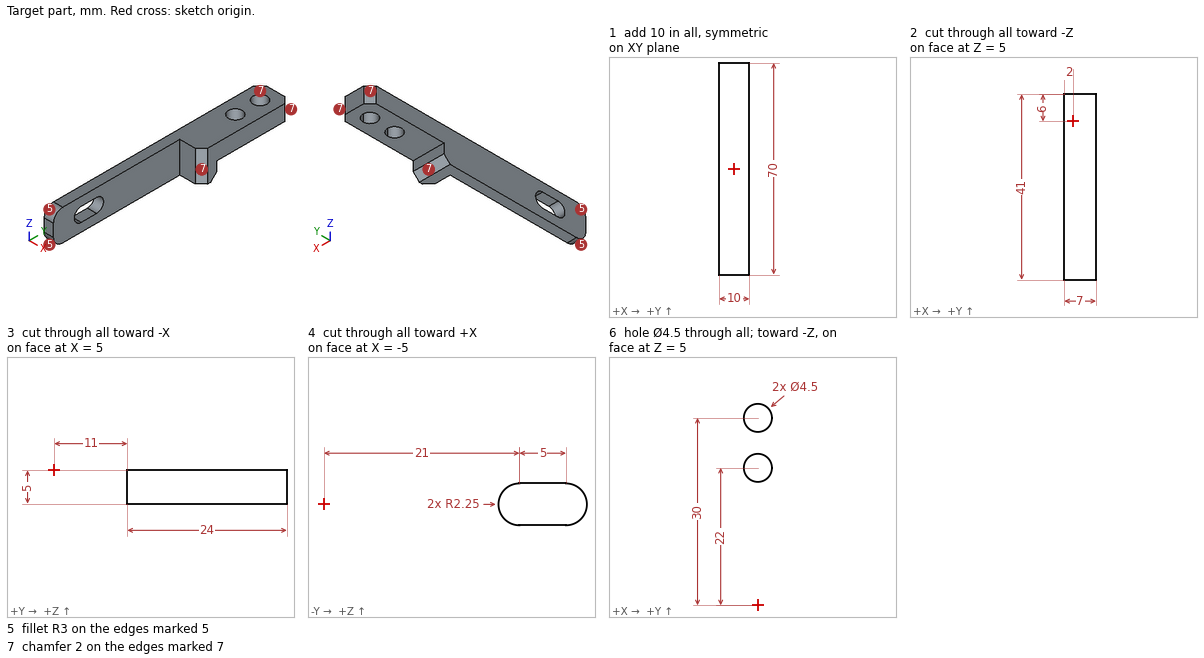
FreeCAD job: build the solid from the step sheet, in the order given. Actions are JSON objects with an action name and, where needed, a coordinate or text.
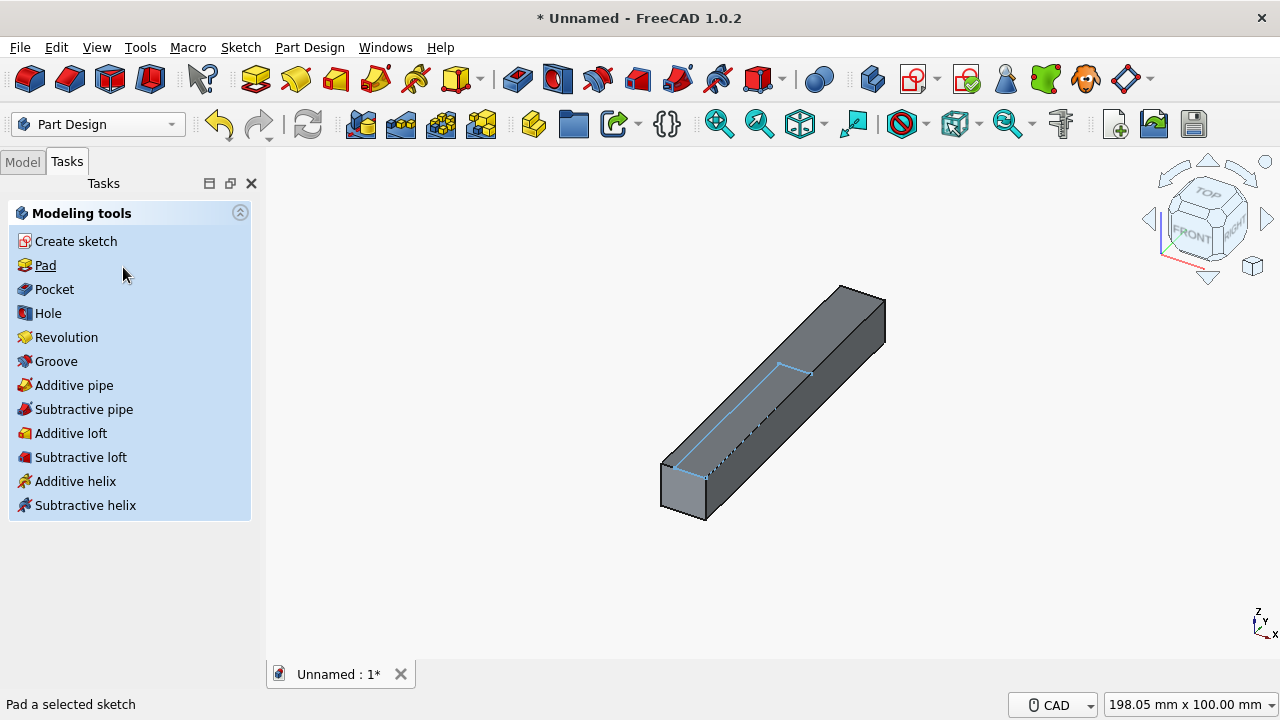
{"action": "left_click", "coordinate": [518, 80]}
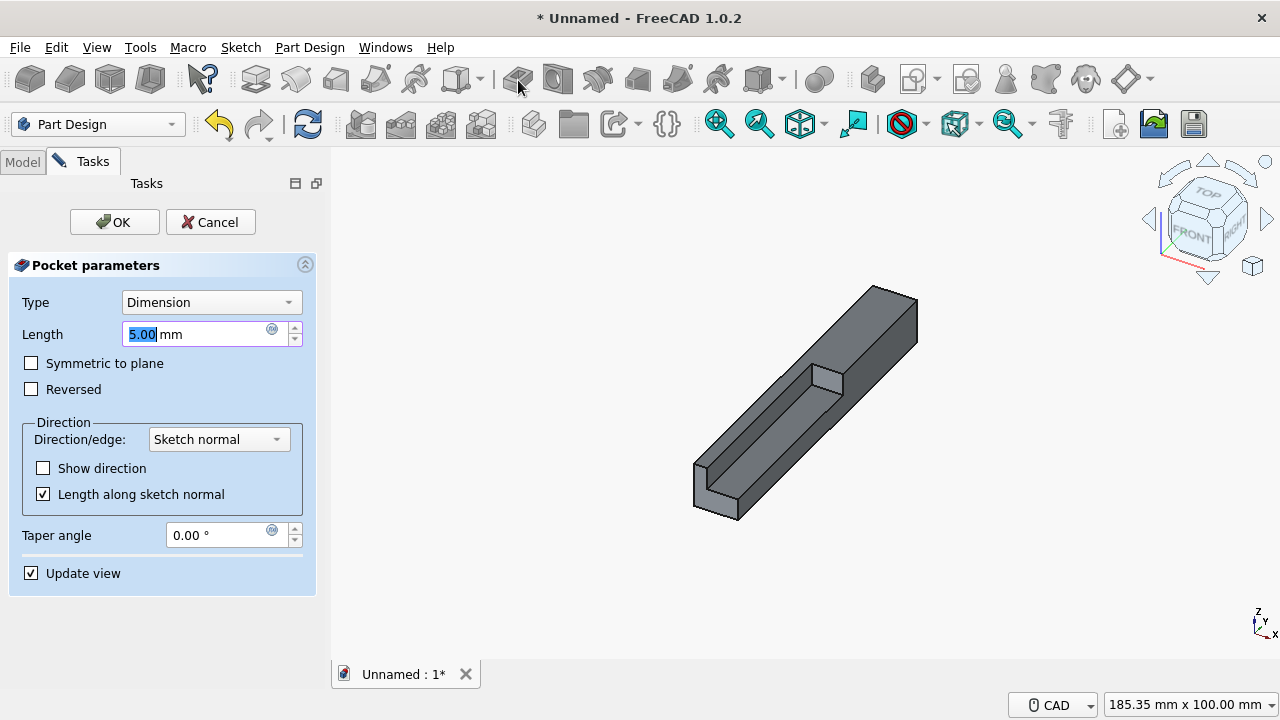
{"action": "left_click", "coordinate": [212, 302]}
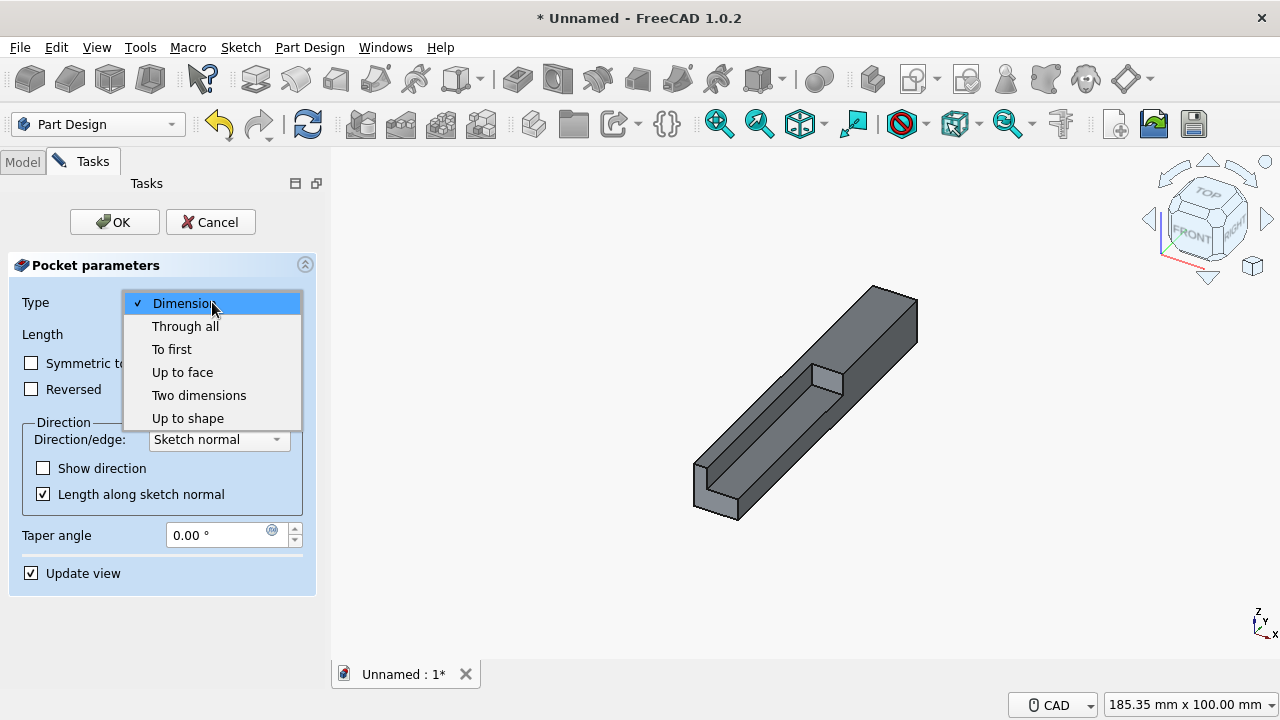
{"action": "left_click", "coordinate": [212, 326]}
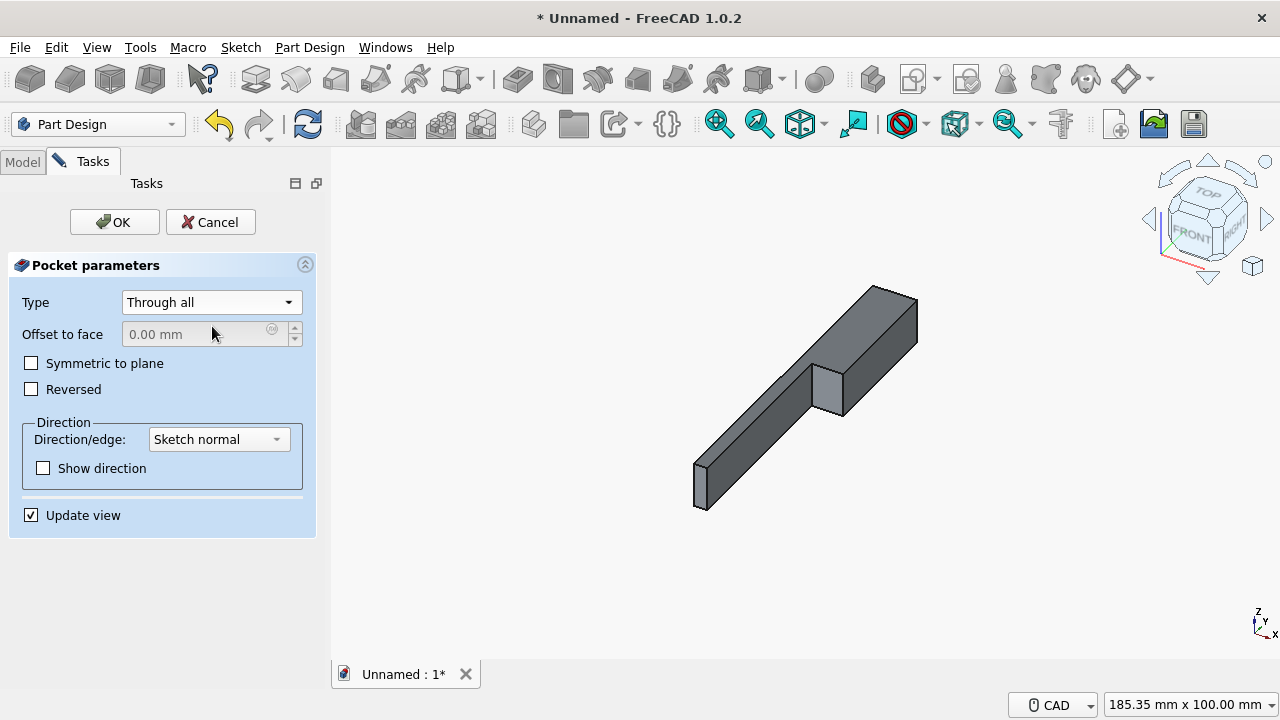
{"action": "left_click", "coordinate": [115, 222]}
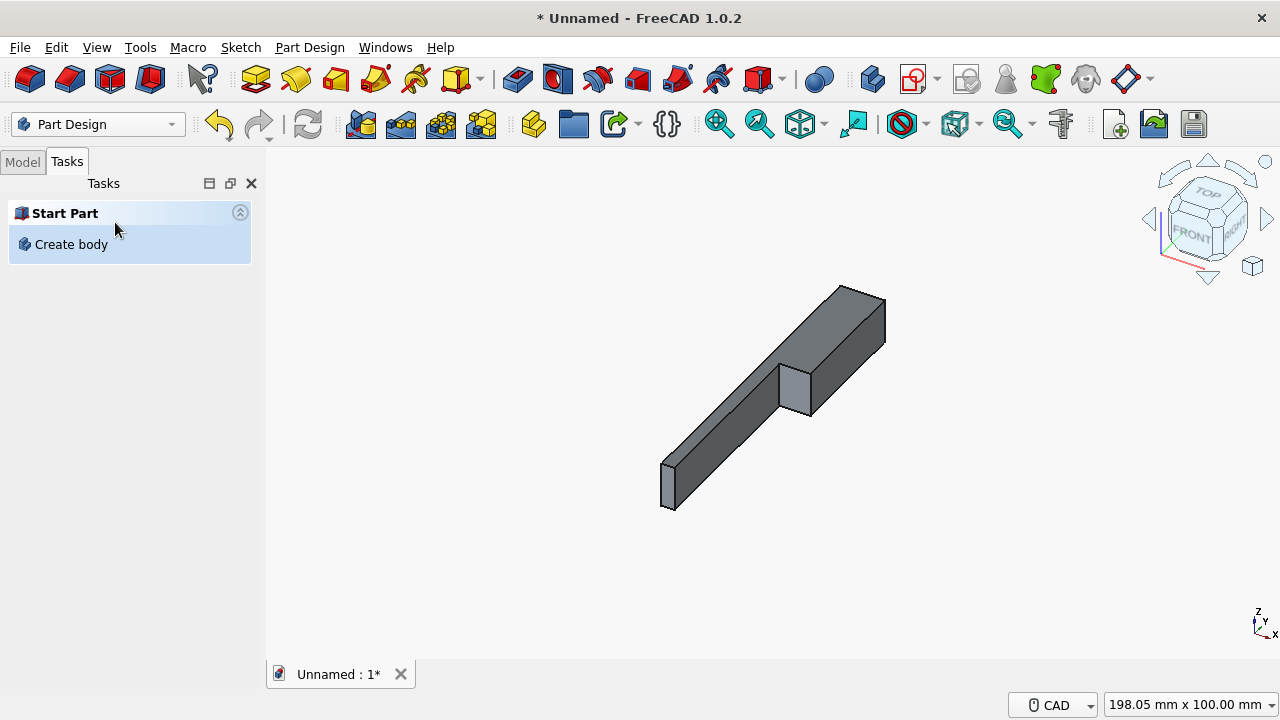
{"action": "left_click", "coordinate": [869, 336]}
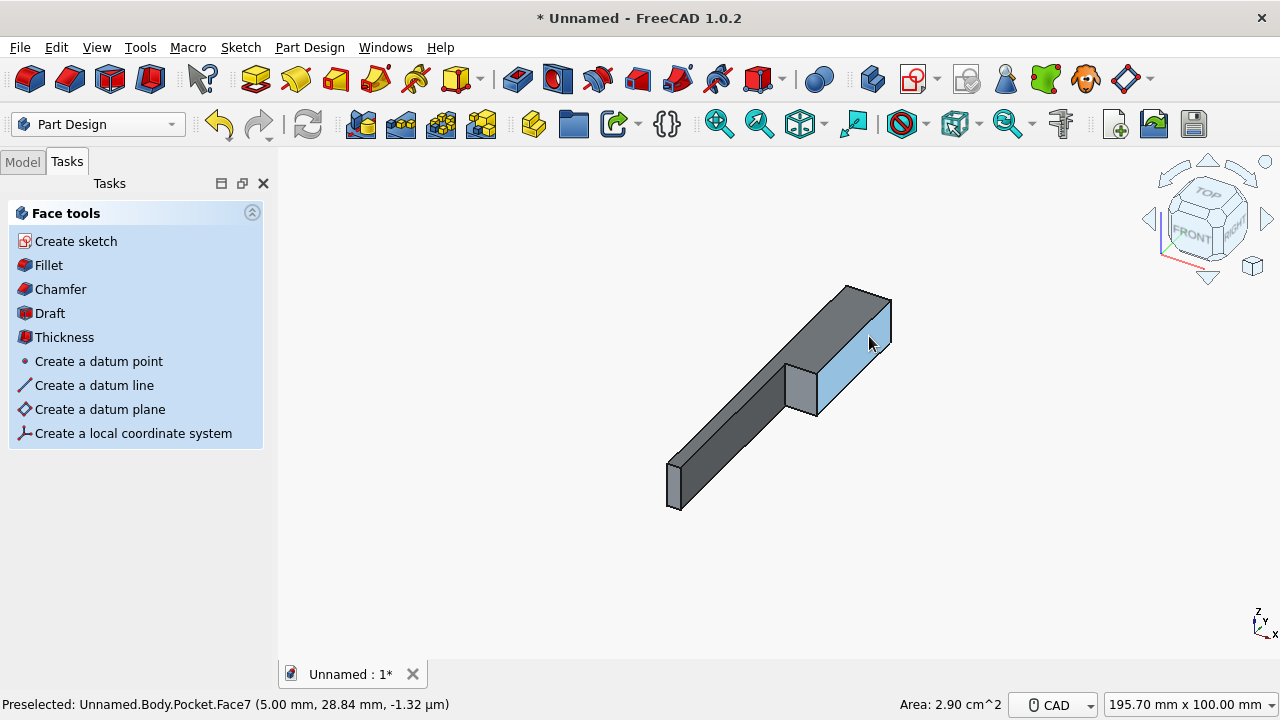
{"action": "left_click", "coordinate": [914, 80]}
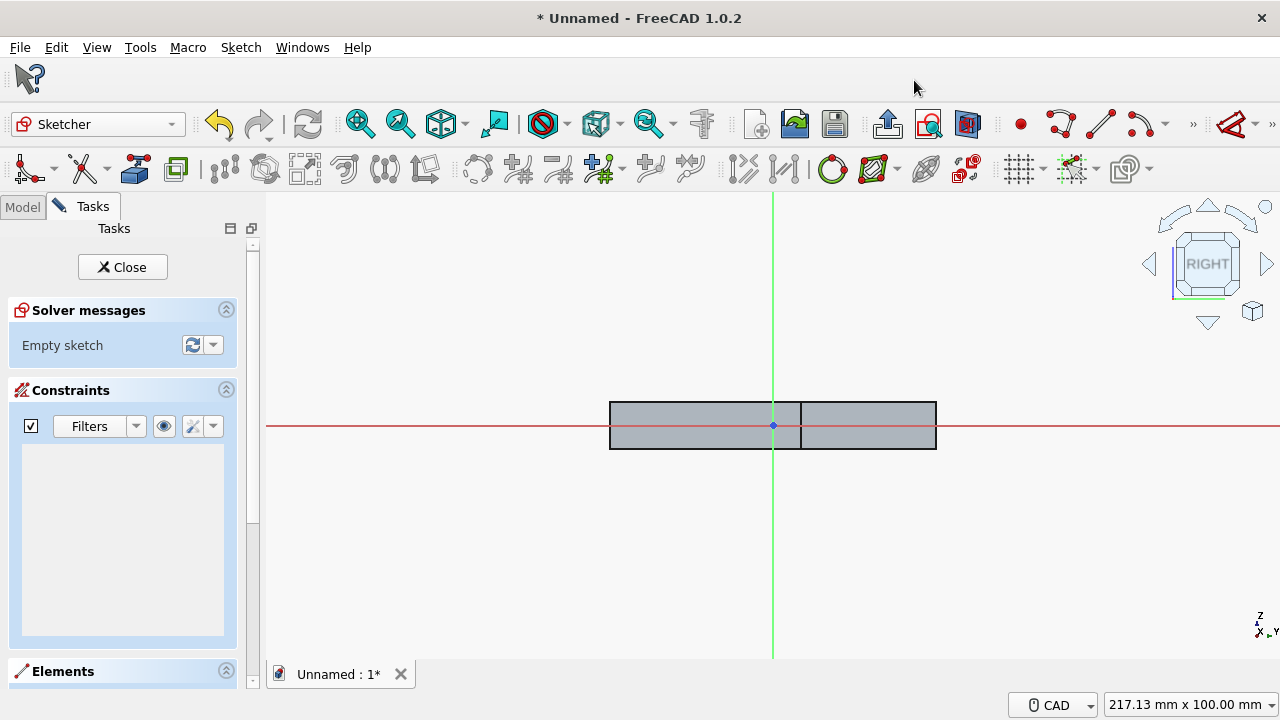
{"action": "scroll", "coordinate": [919, 442], "scroll_direction": "up", "scroll_amount": 6}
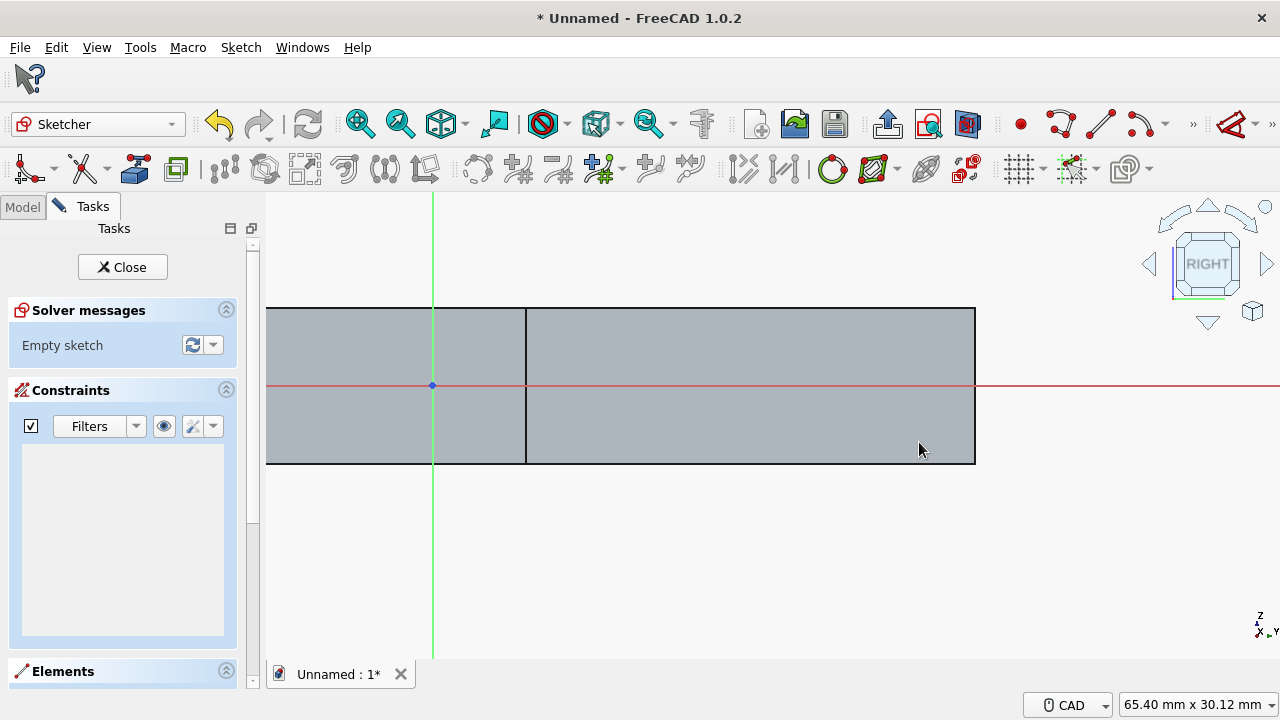
{"action": "key", "text": "g r"}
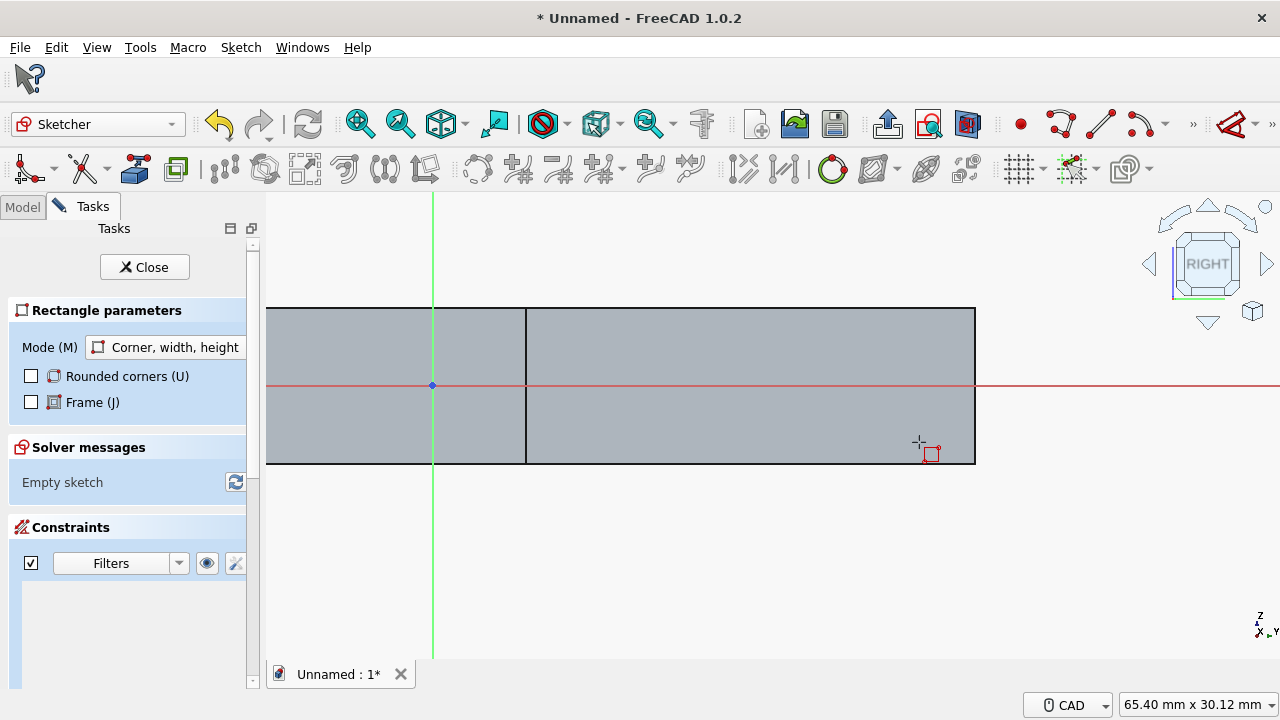
{"action": "left_click", "coordinate": [603, 386]}
{"action": "left_click", "coordinate": [975, 463]}
{"action": "key", "text": "Escape"}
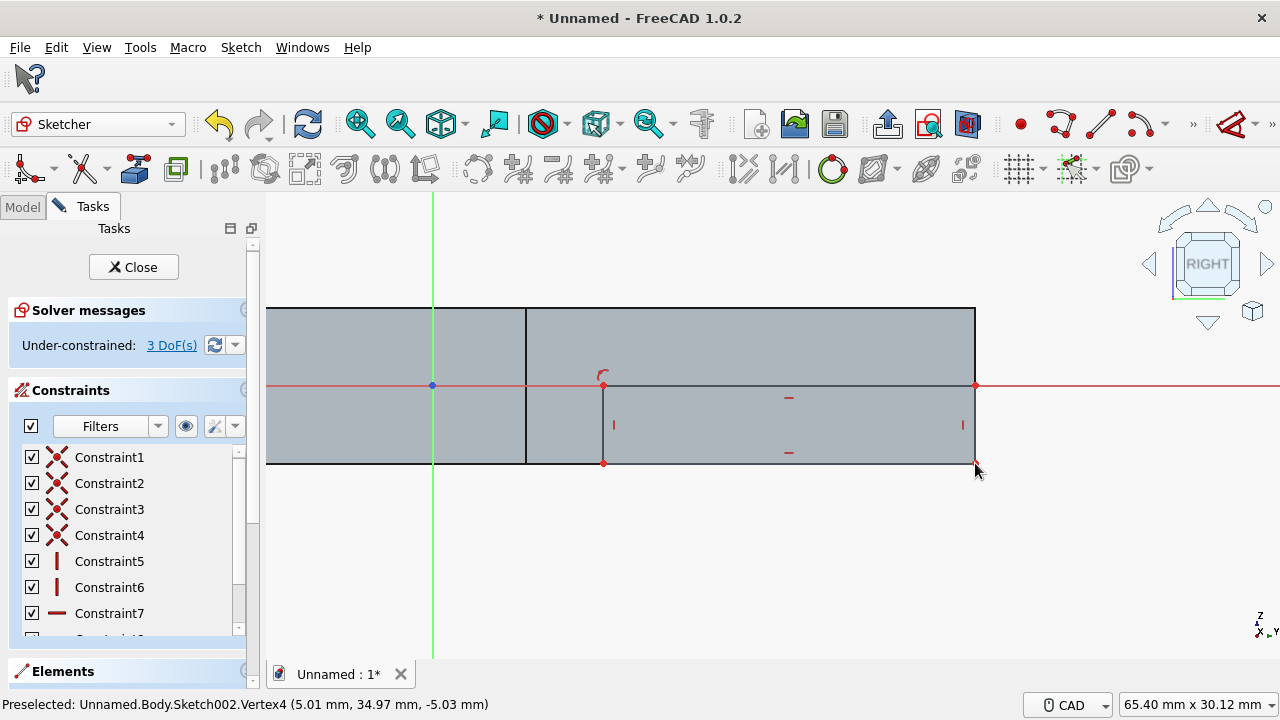
{"action": "left_click", "coordinate": [1232, 124]}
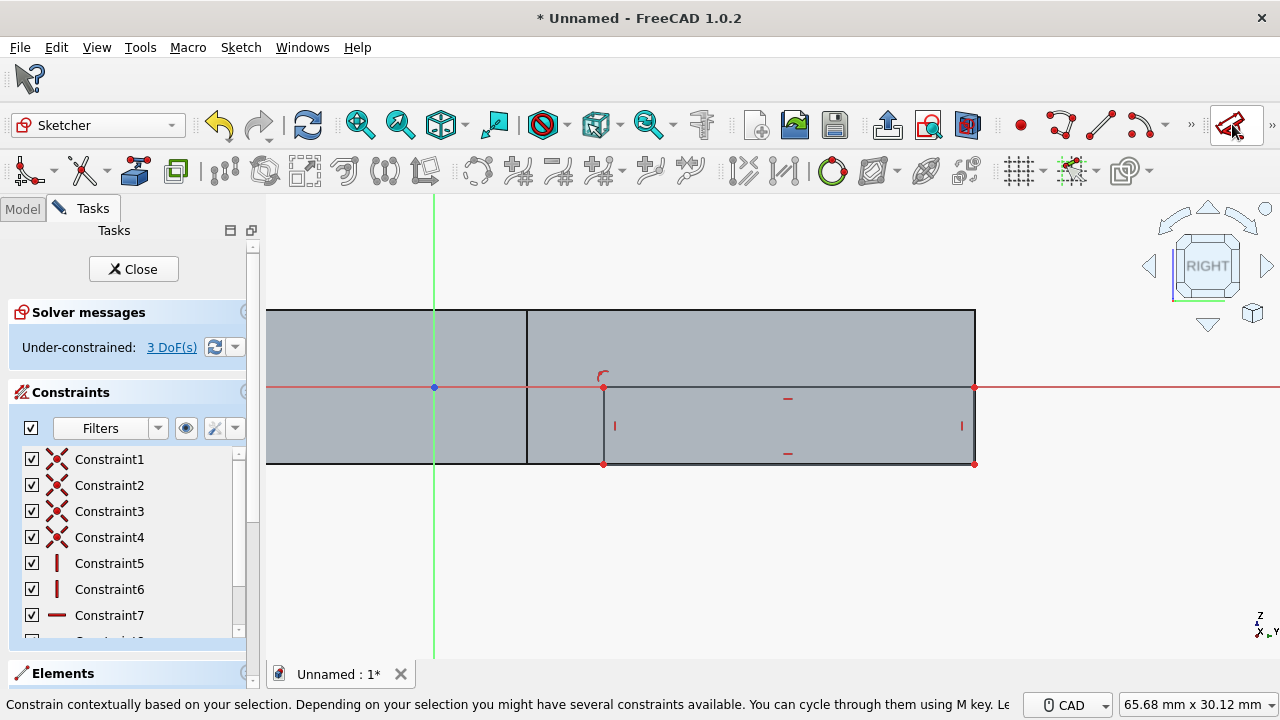
{"action": "left_click", "coordinate": [604, 410]}
{"action": "left_click", "coordinate": [570, 426]}